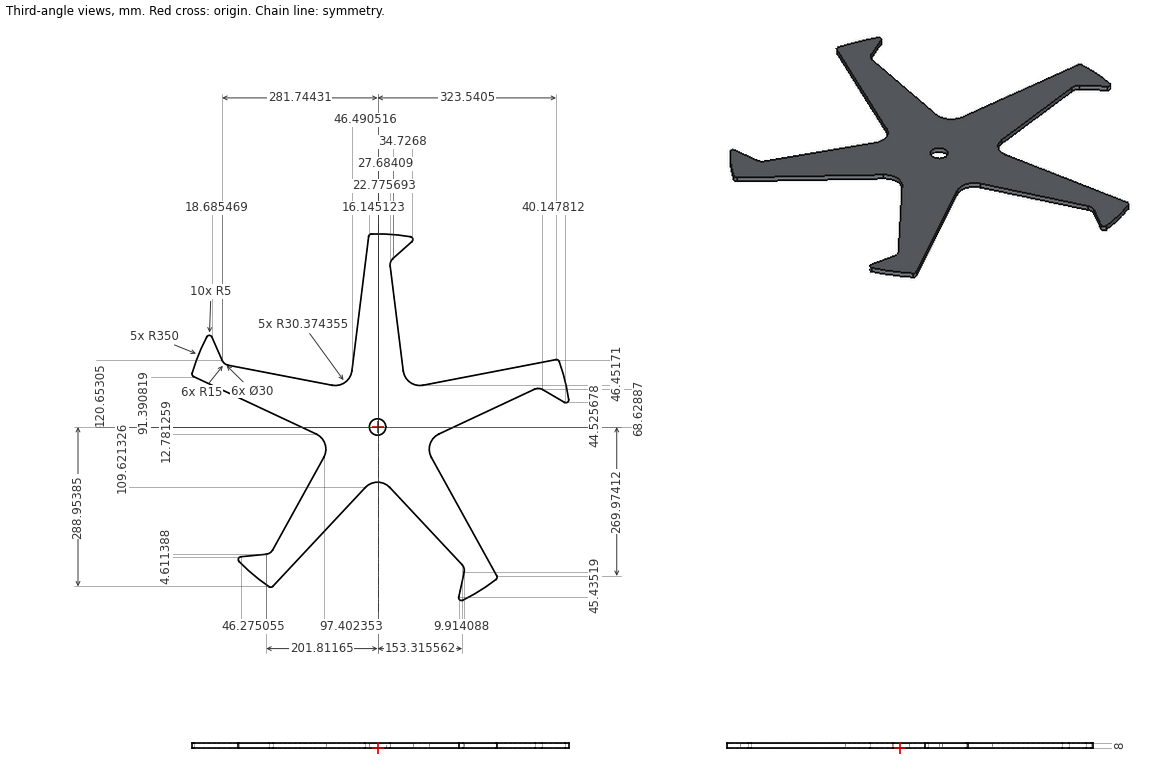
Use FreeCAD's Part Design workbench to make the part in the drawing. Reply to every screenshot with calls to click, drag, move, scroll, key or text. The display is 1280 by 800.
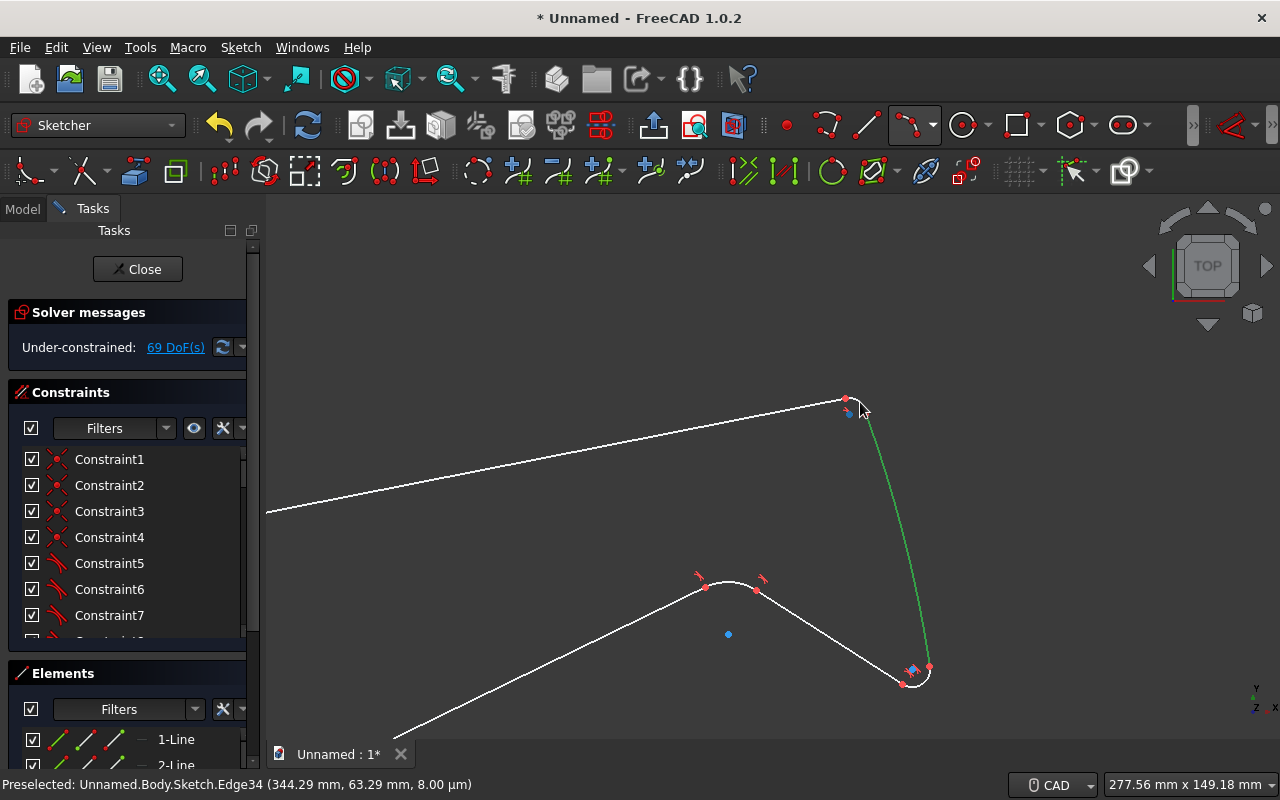
click(859, 402)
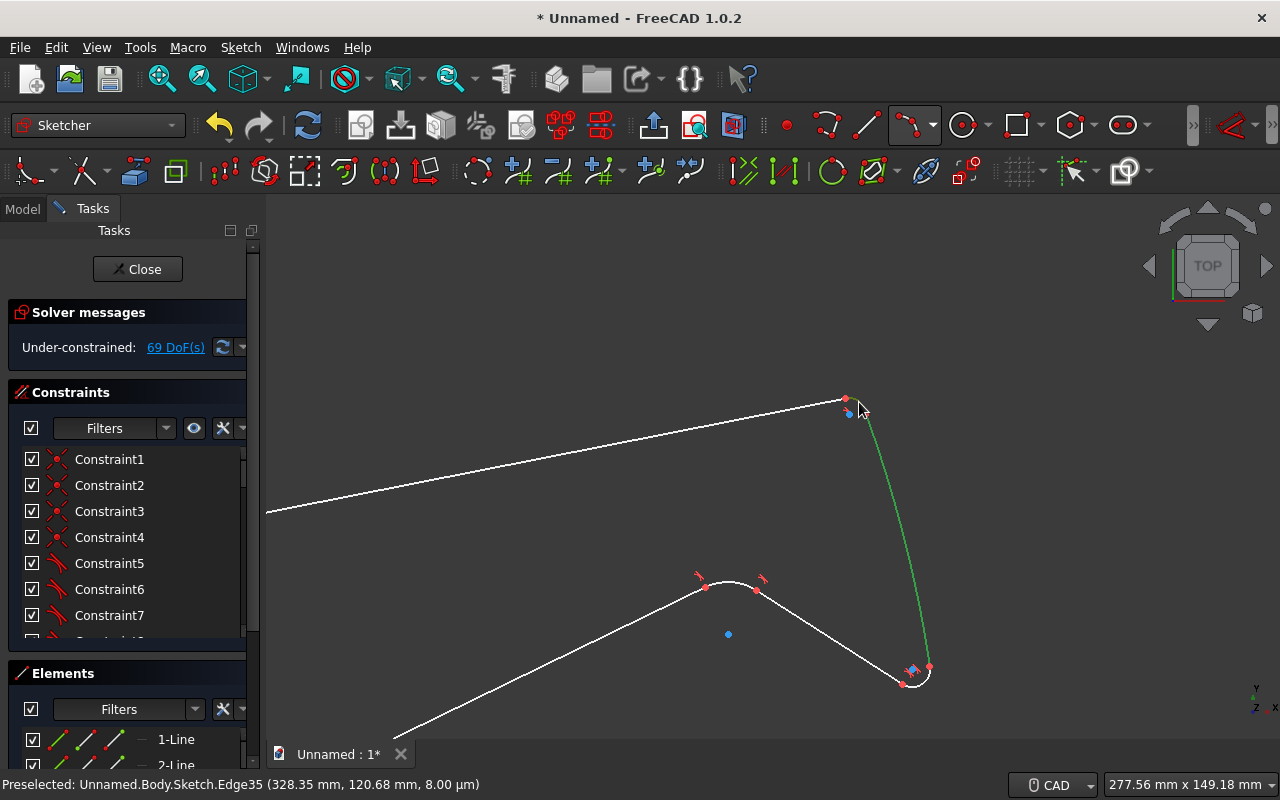
key(t)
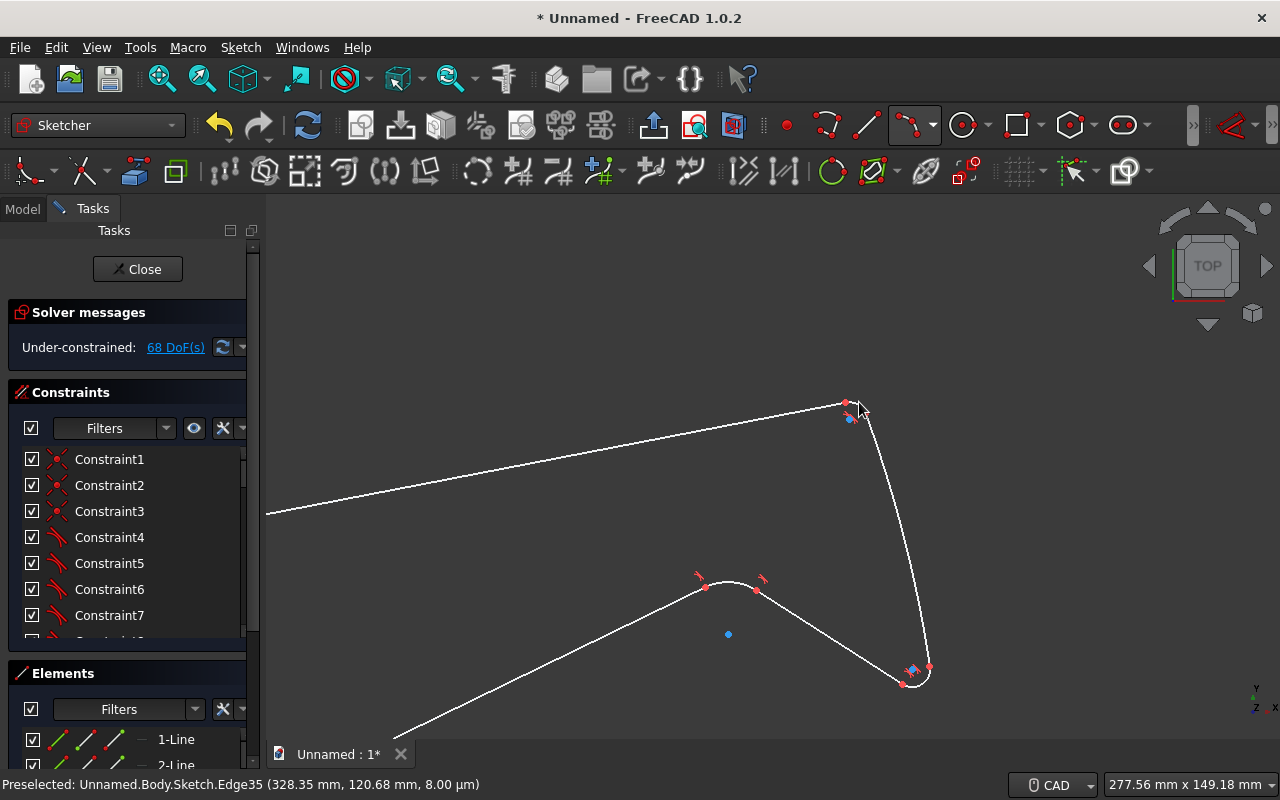
scroll(865, 417, down, 10)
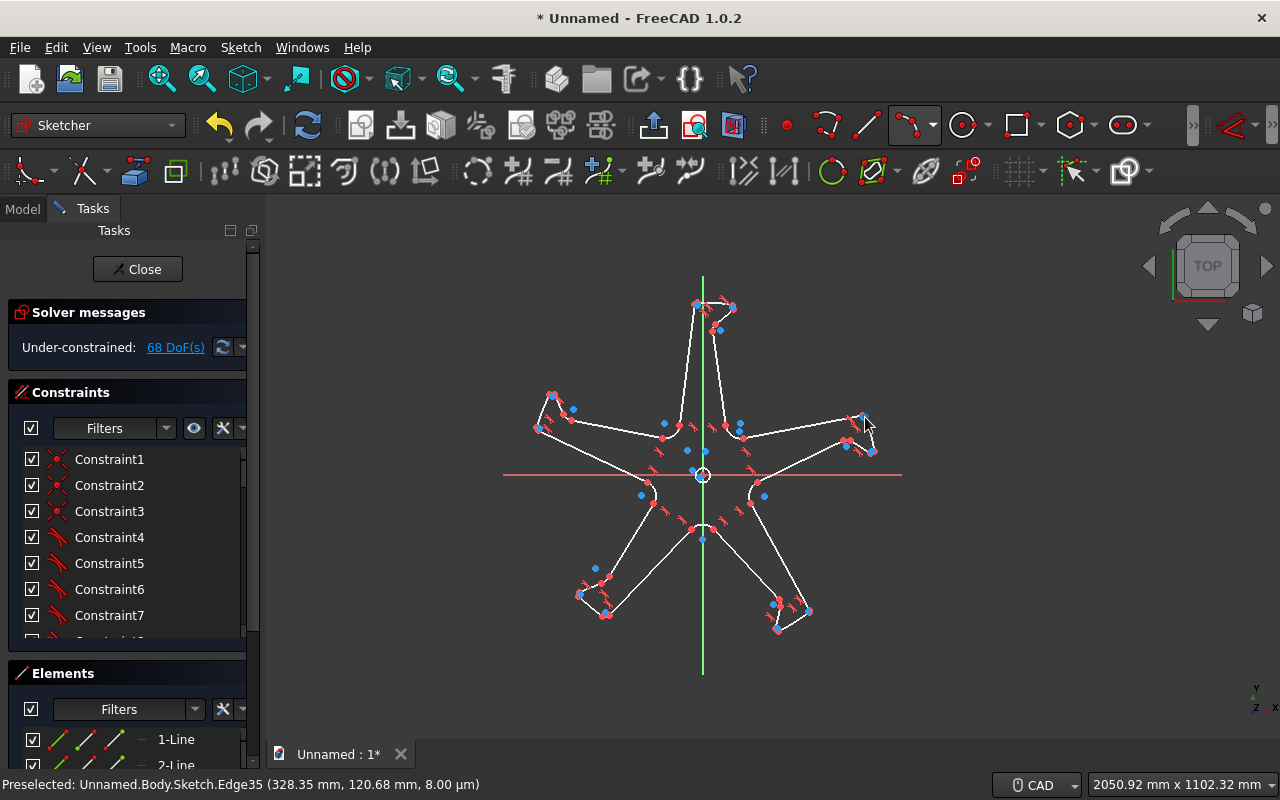
scroll(735, 308, up, 11)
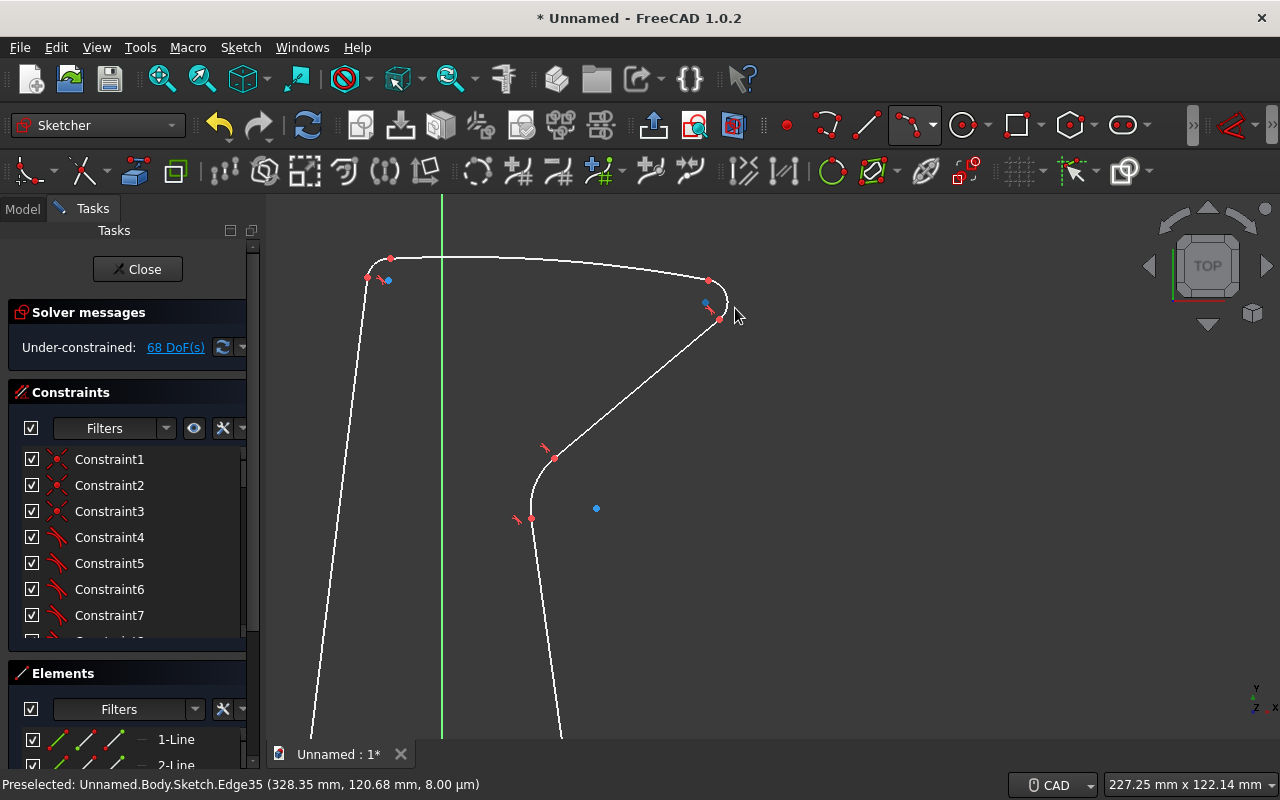
click(727, 307)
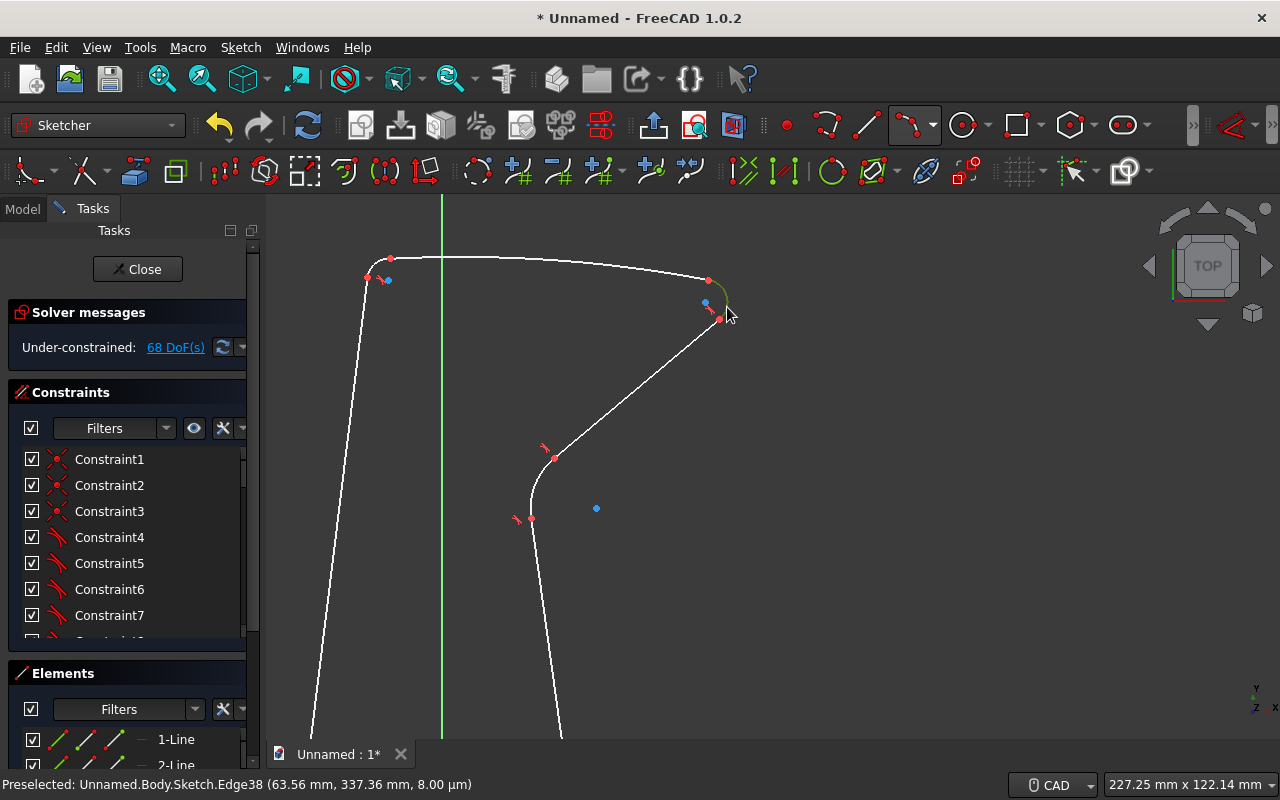
scroll(734, 308, down, 11)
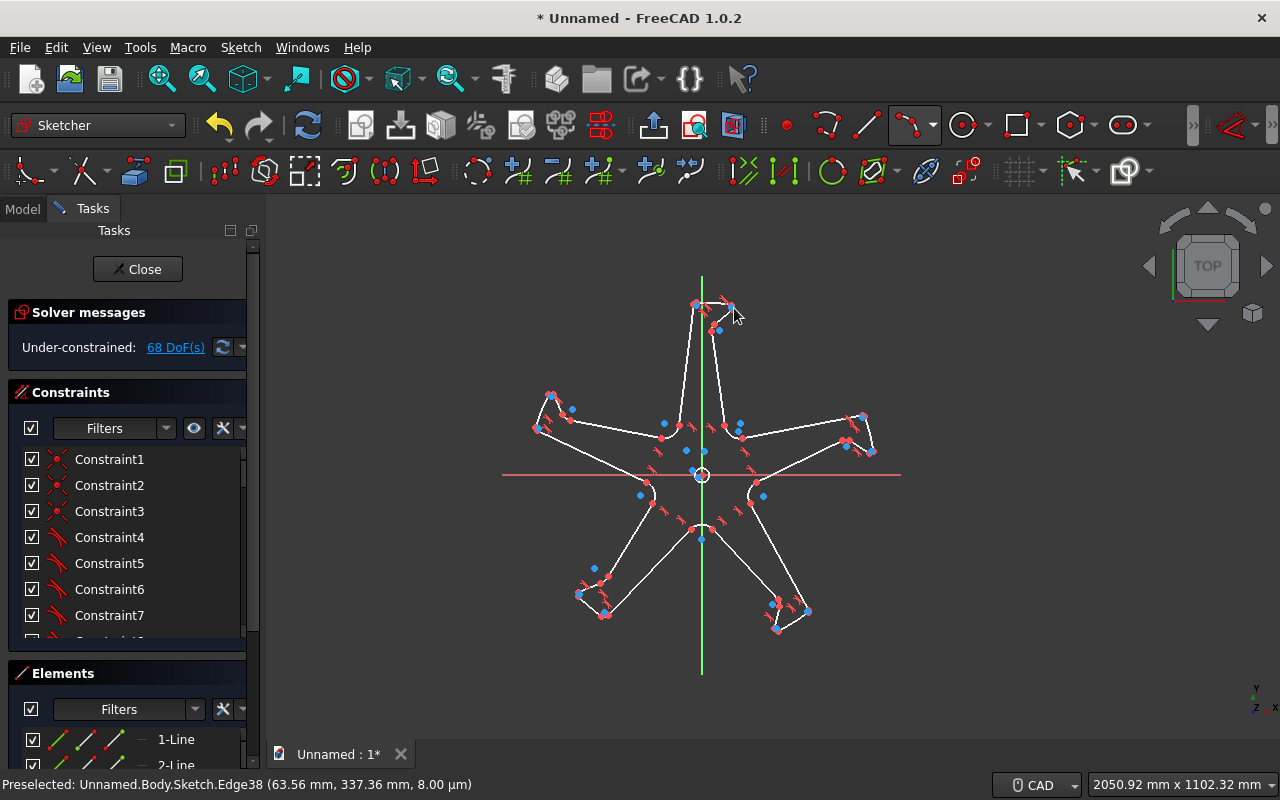
scroll(721, 304, up, 2)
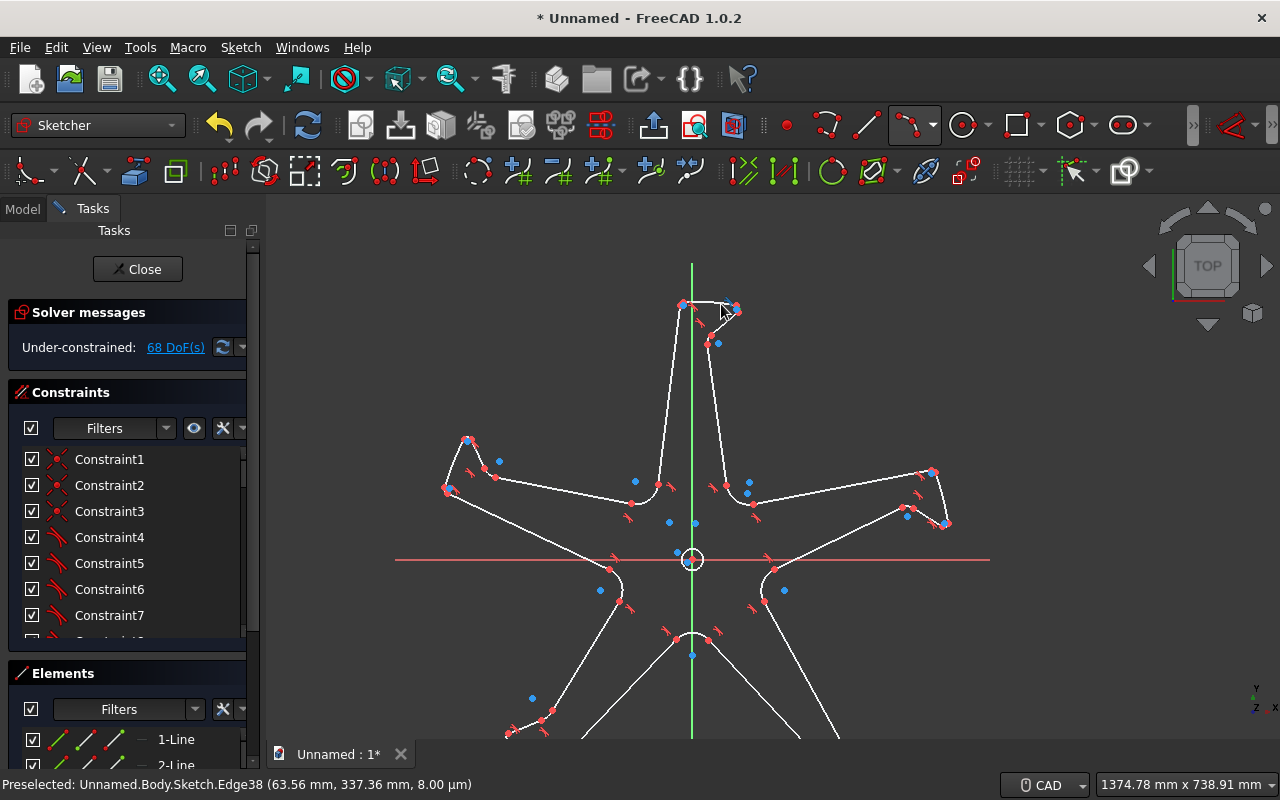
click(721, 303)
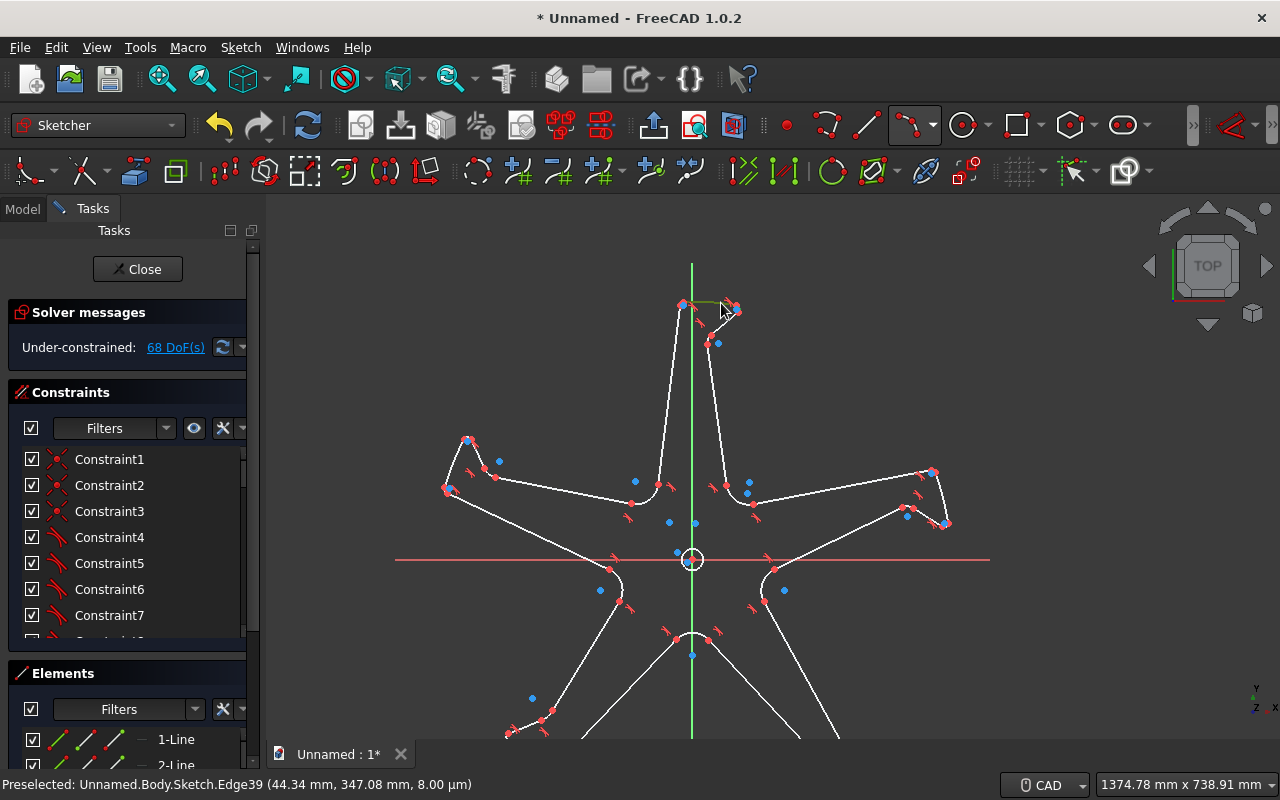
key(t)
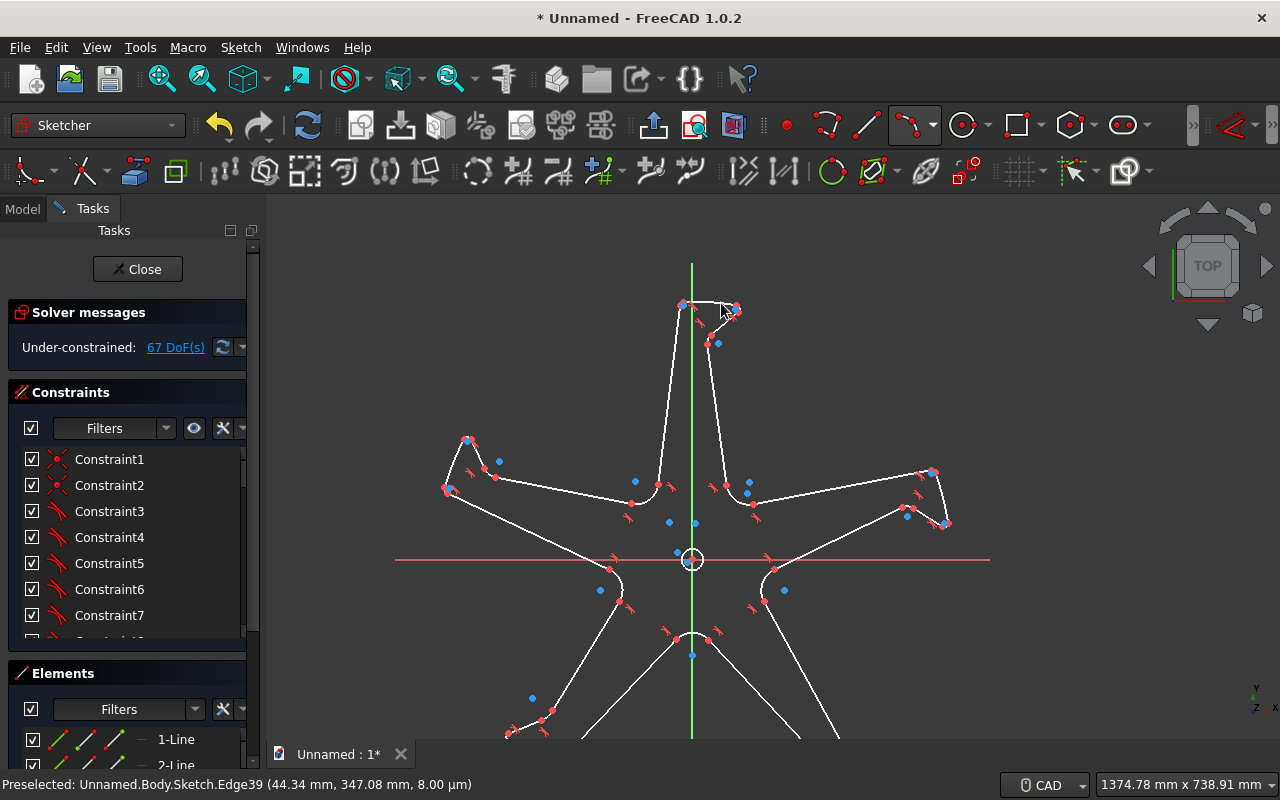
click(721, 303)